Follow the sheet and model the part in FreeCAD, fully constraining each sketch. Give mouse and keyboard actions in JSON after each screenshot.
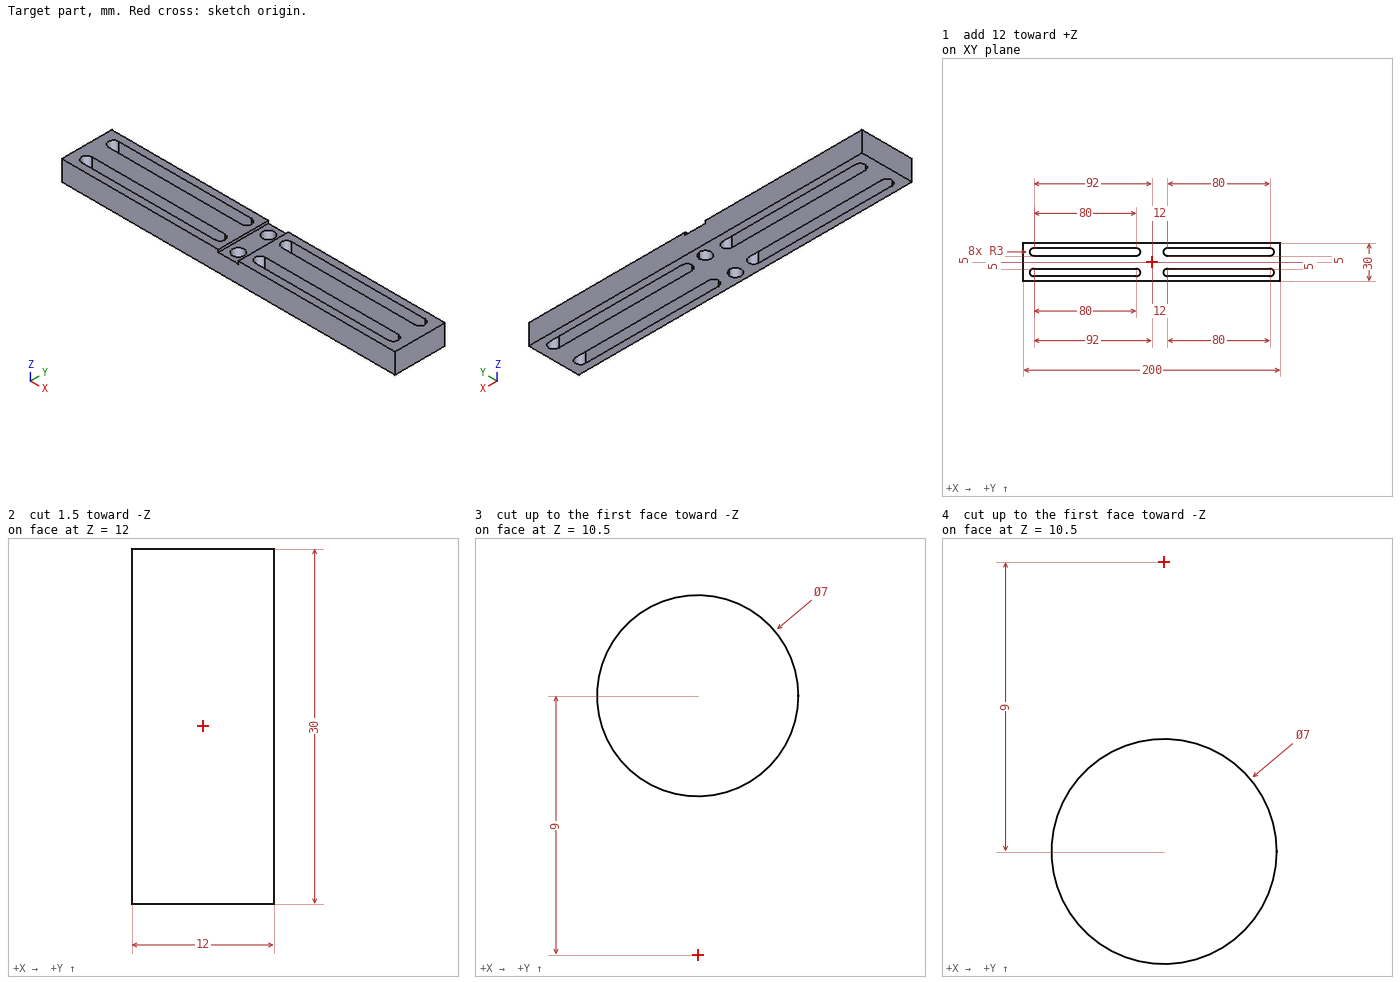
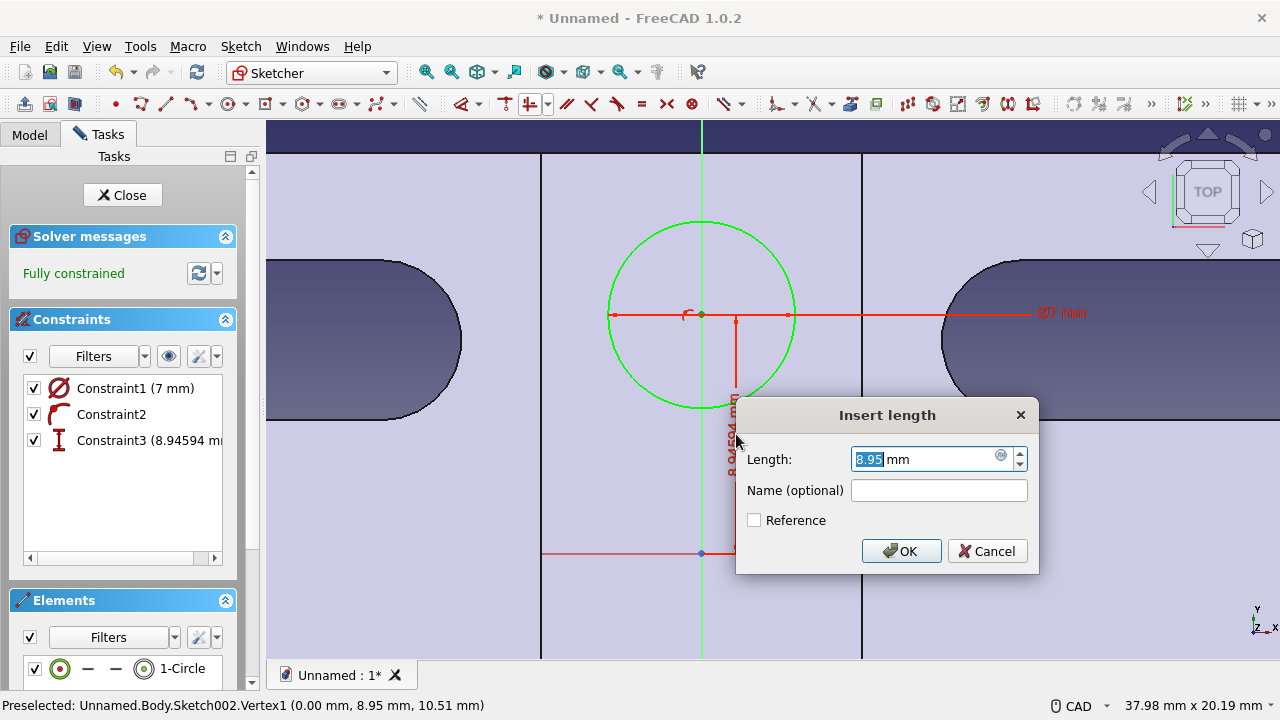
{"action": "type", "text": "9"}
{"action": "key", "text": "Return"}
{"action": "key", "text": "Escape"}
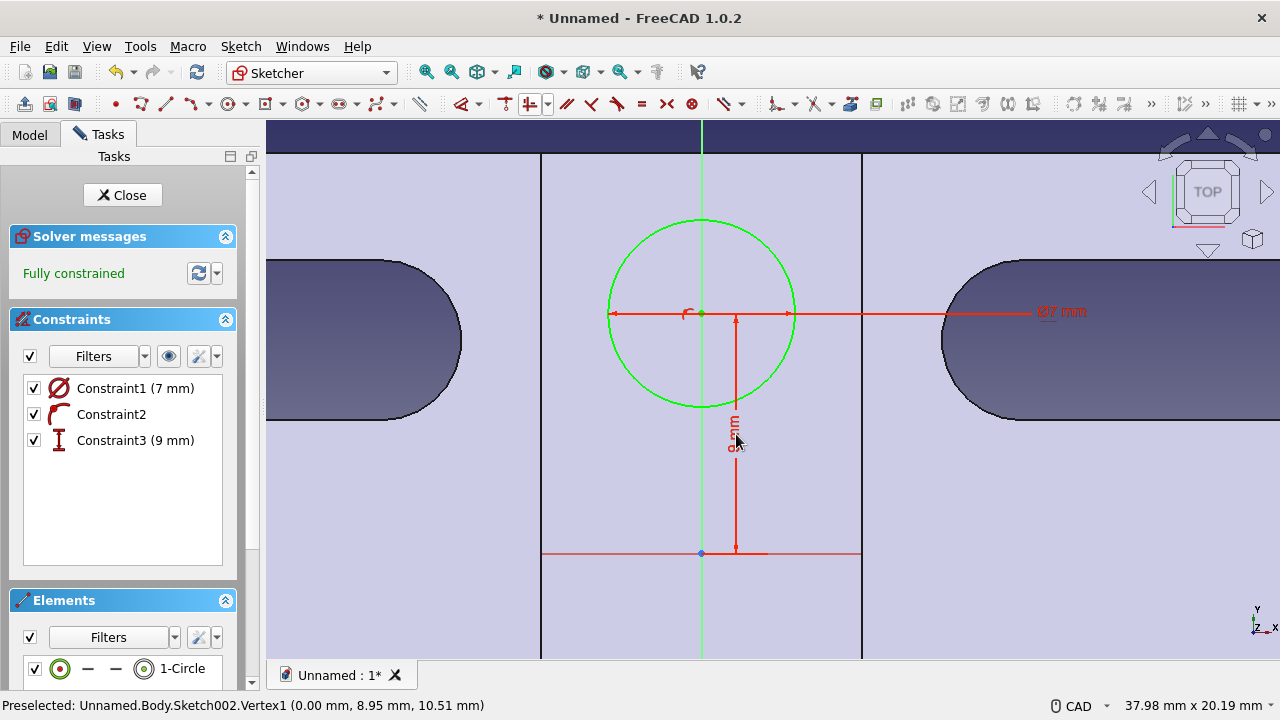
{"action": "left_click", "coordinate": [123, 195]}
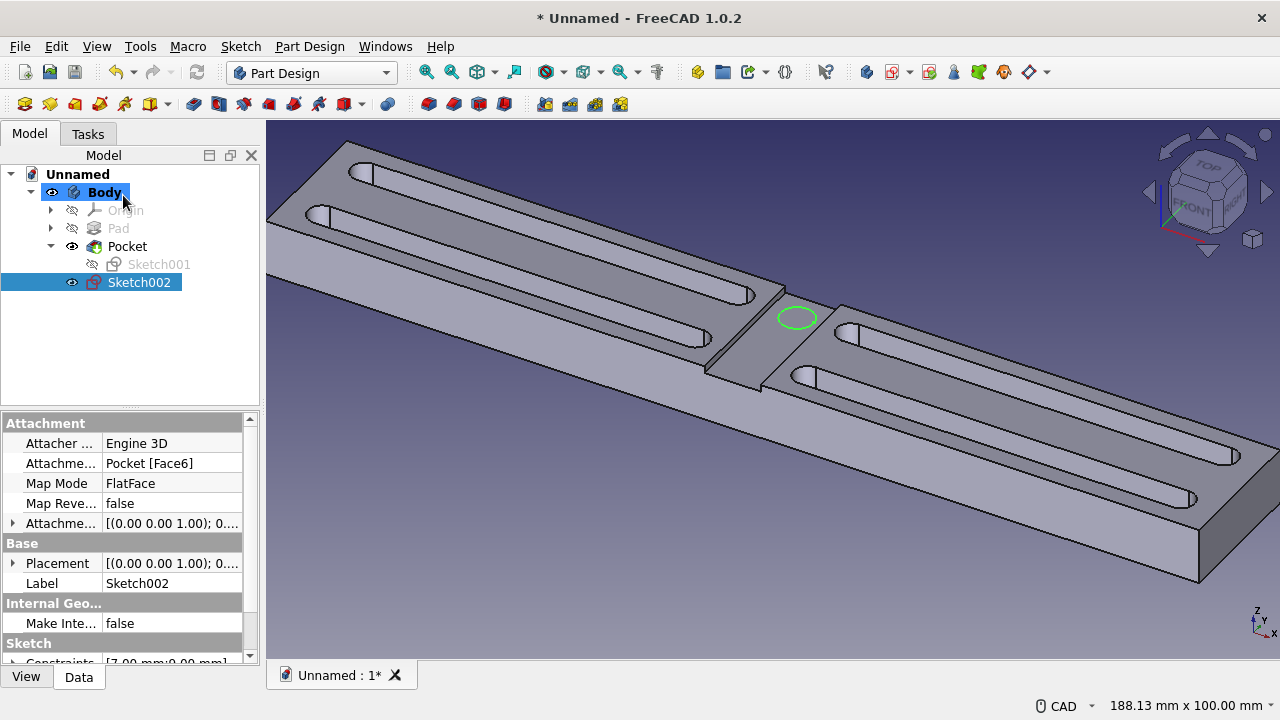
{"action": "left_click", "coordinate": [194, 104]}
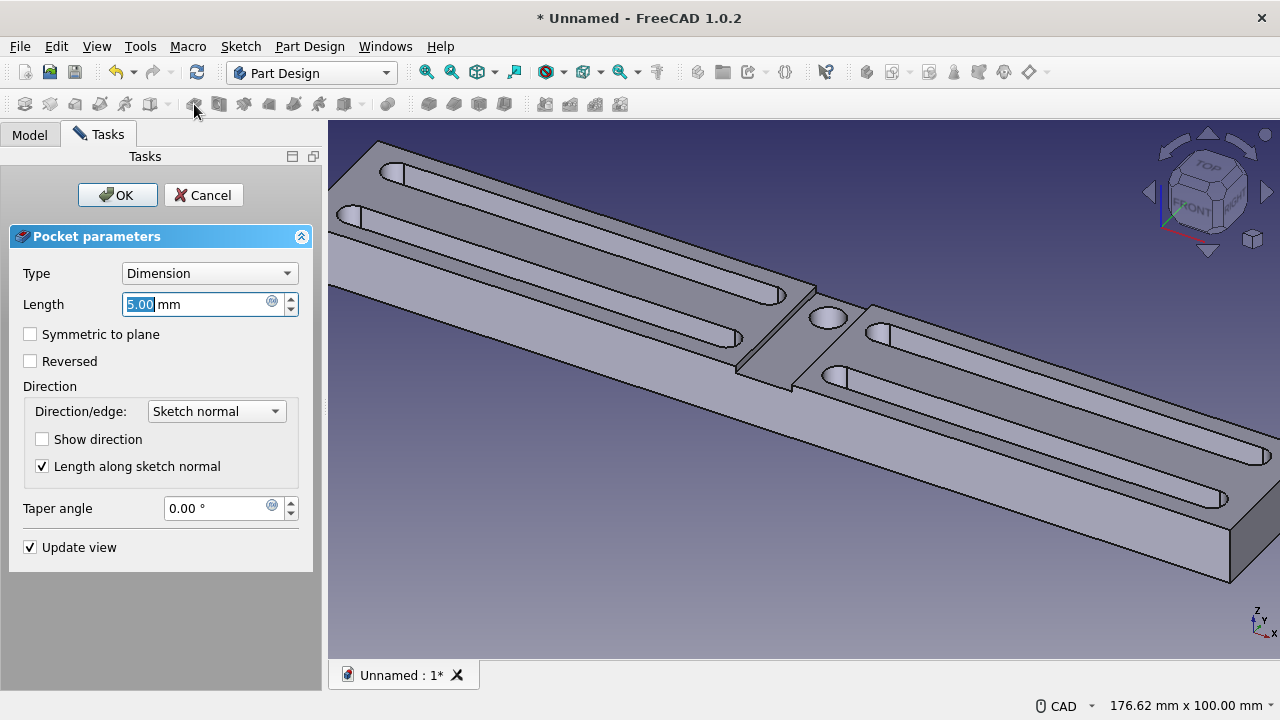
{"action": "left_click", "coordinate": [210, 274]}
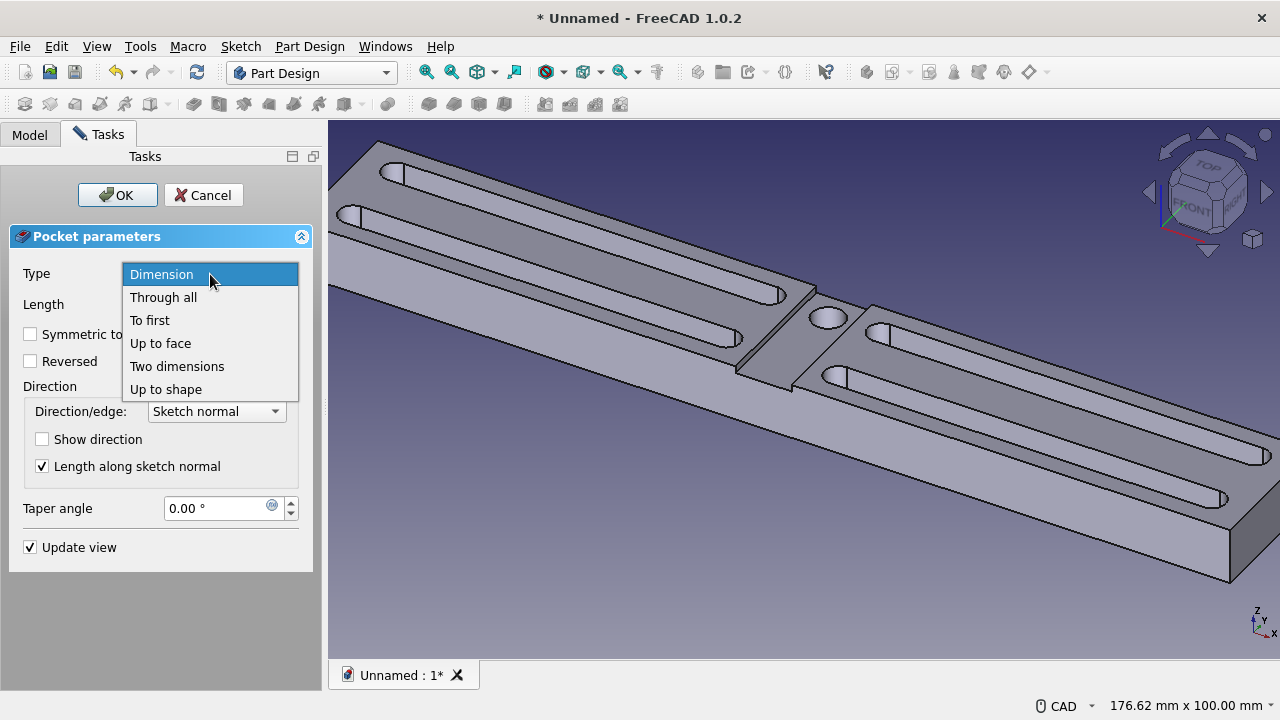
{"action": "left_click", "coordinate": [208, 320]}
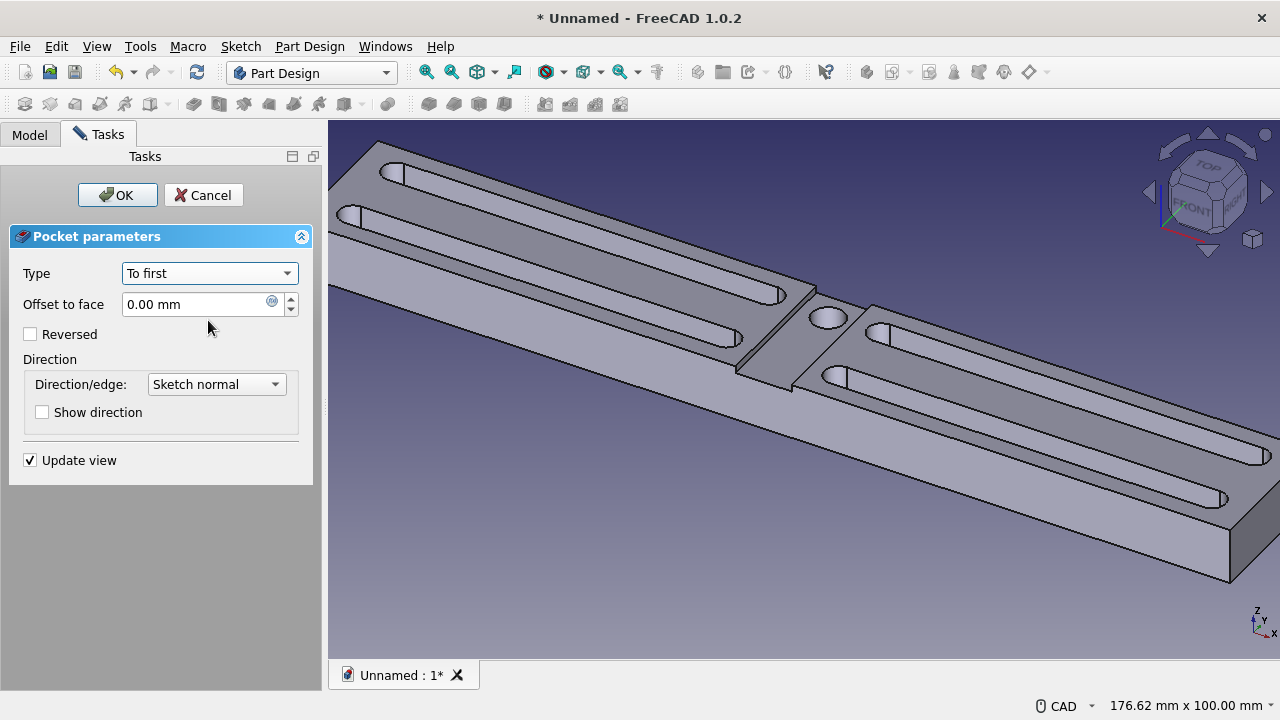
{"action": "left_click", "coordinate": [118, 195]}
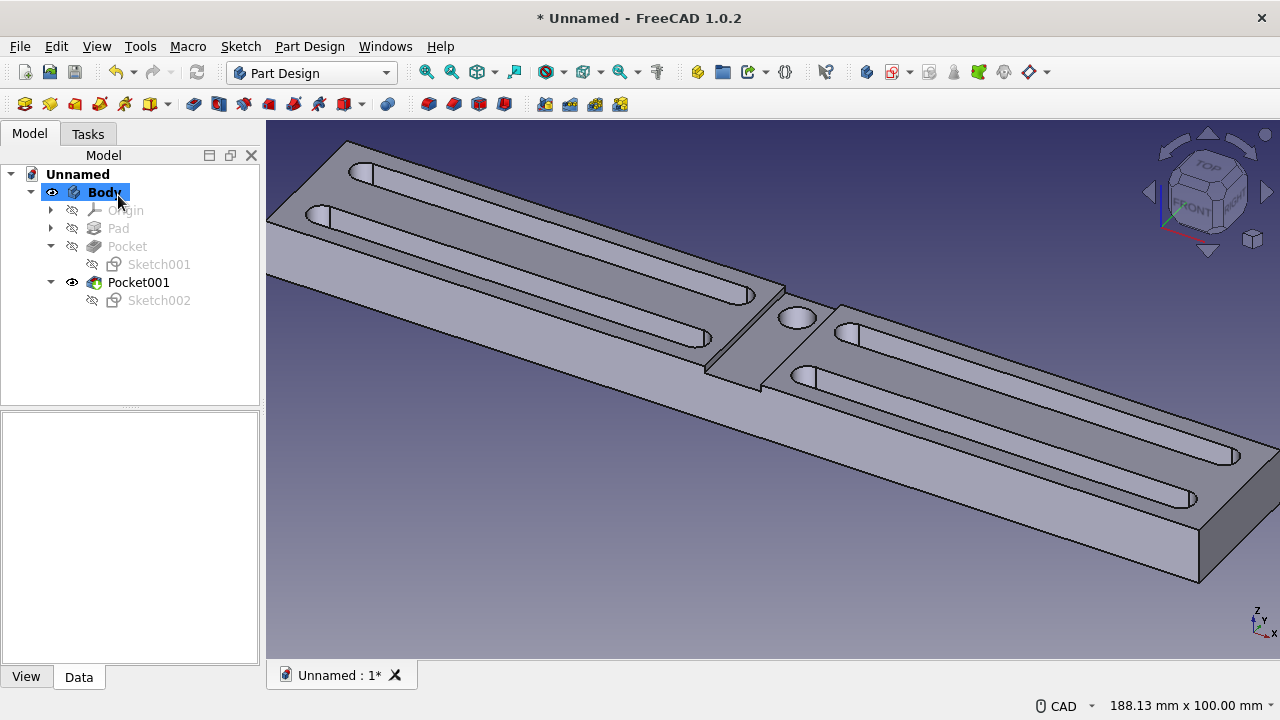
{"action": "left_click", "coordinate": [761, 353]}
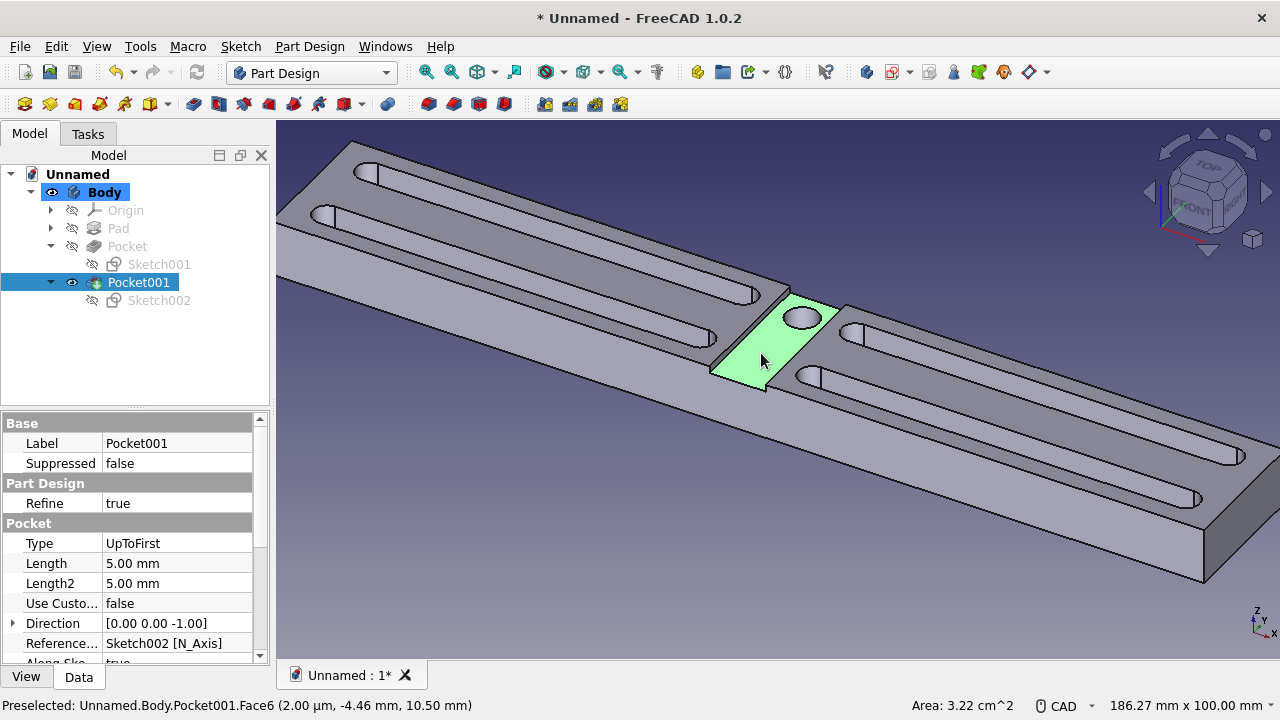
{"action": "left_click", "coordinate": [892, 72]}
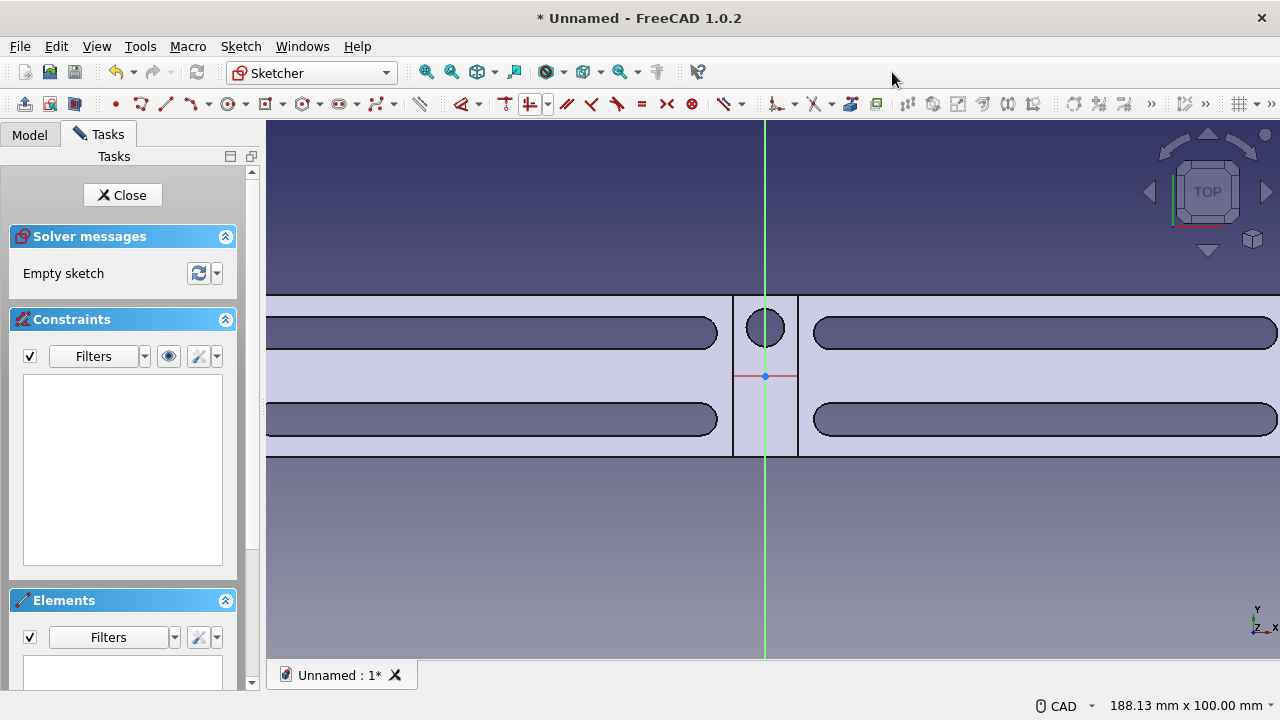
{"action": "left_click", "coordinate": [75, 104]}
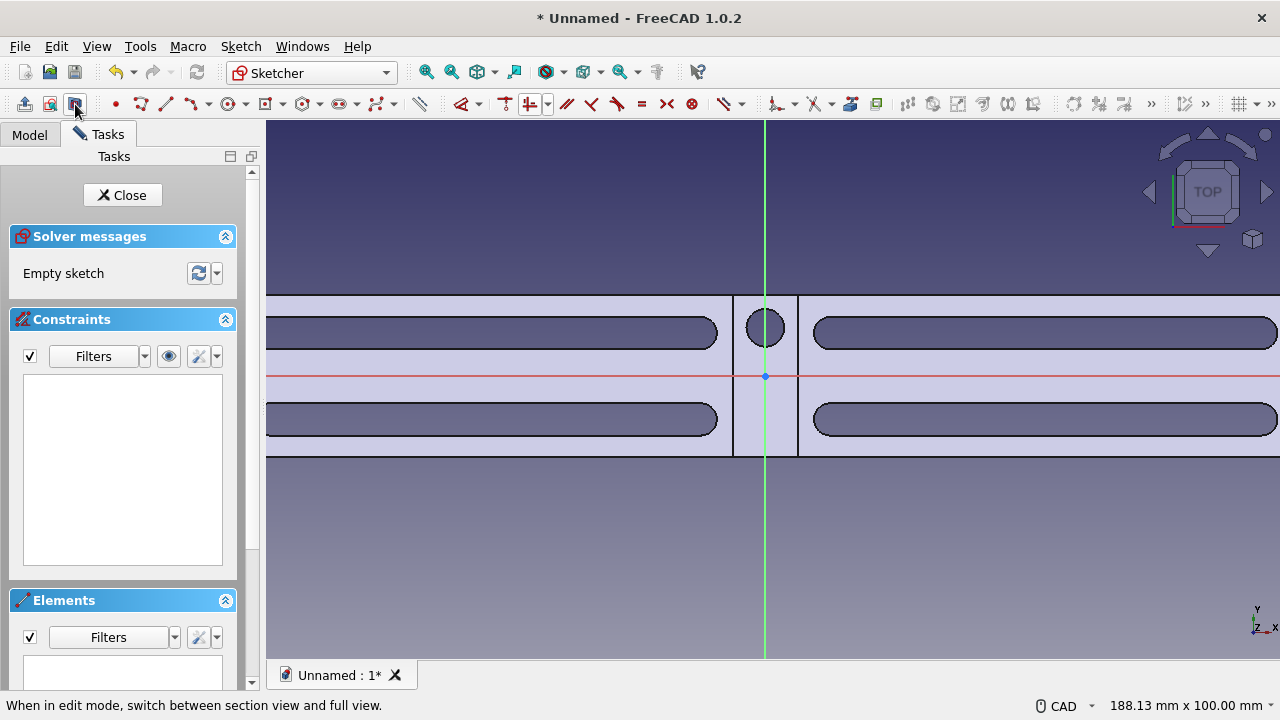
{"action": "scroll", "coordinate": [781, 415], "scroll_direction": "up", "scroll_amount": 8}